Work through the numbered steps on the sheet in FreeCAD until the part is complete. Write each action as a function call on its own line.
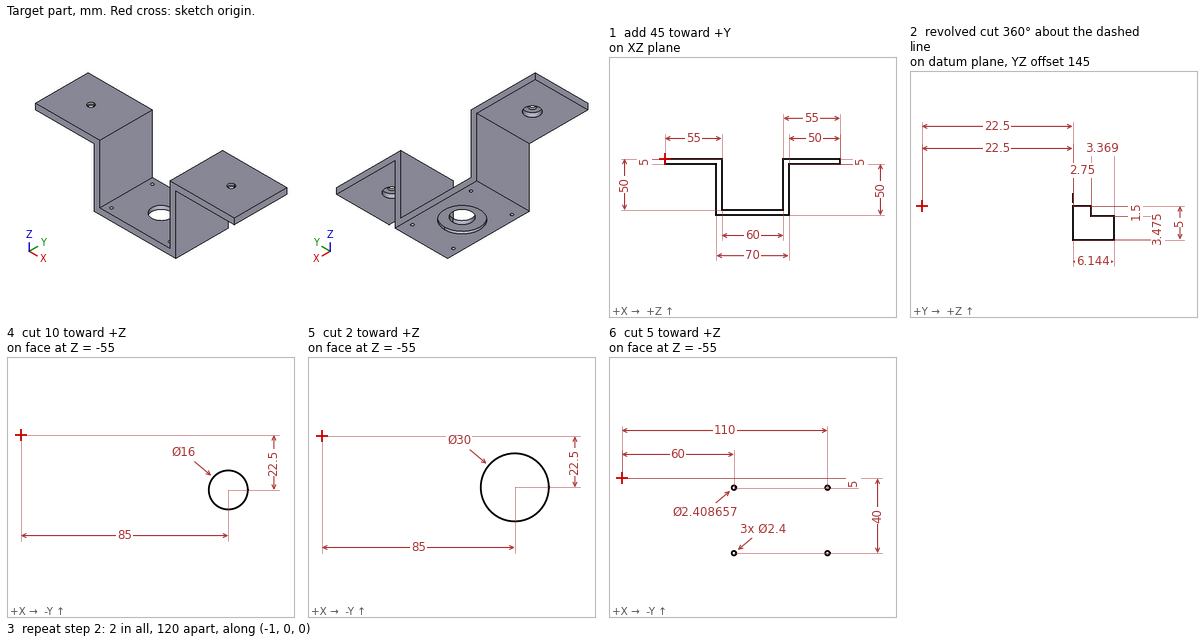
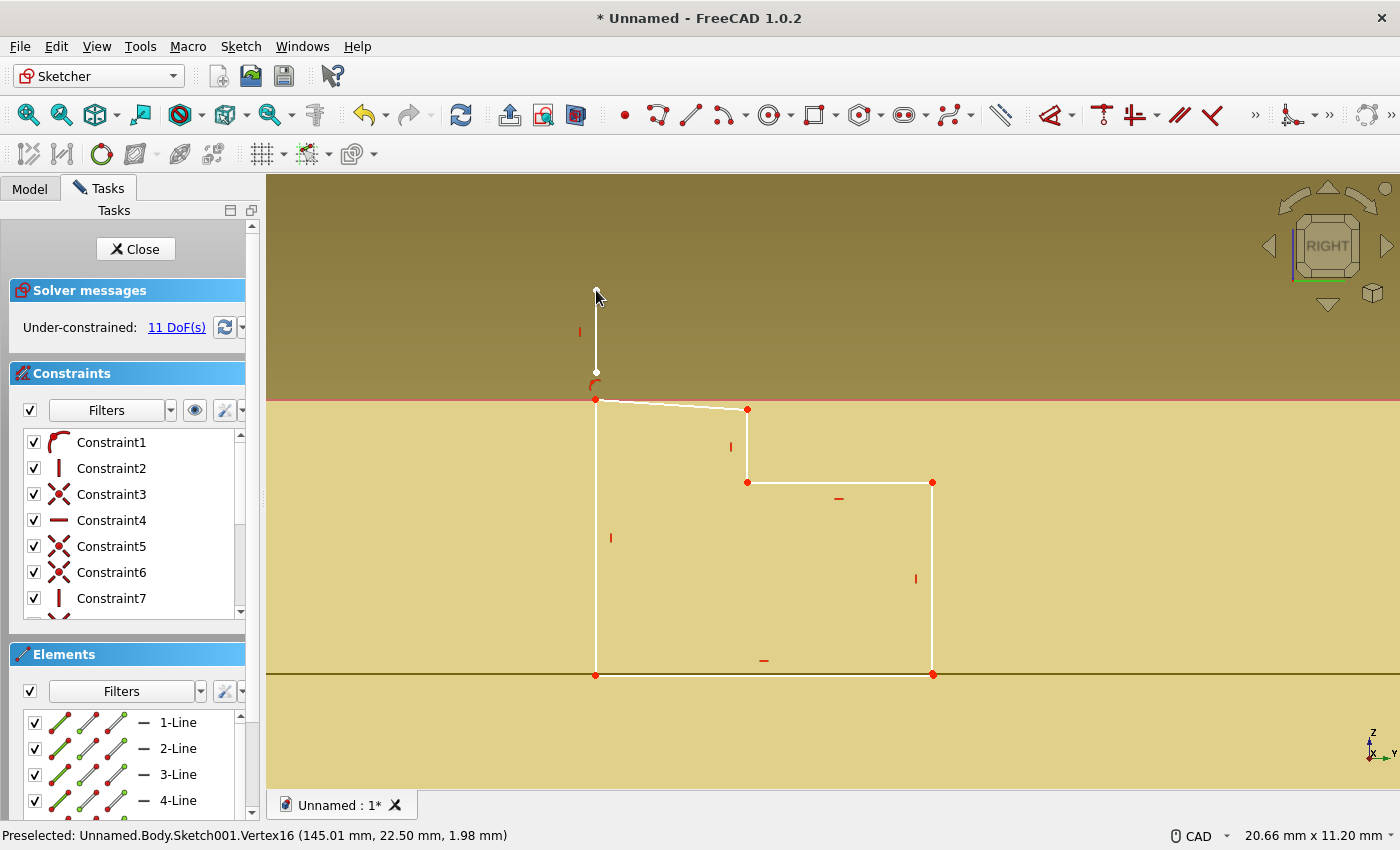
click(596, 348)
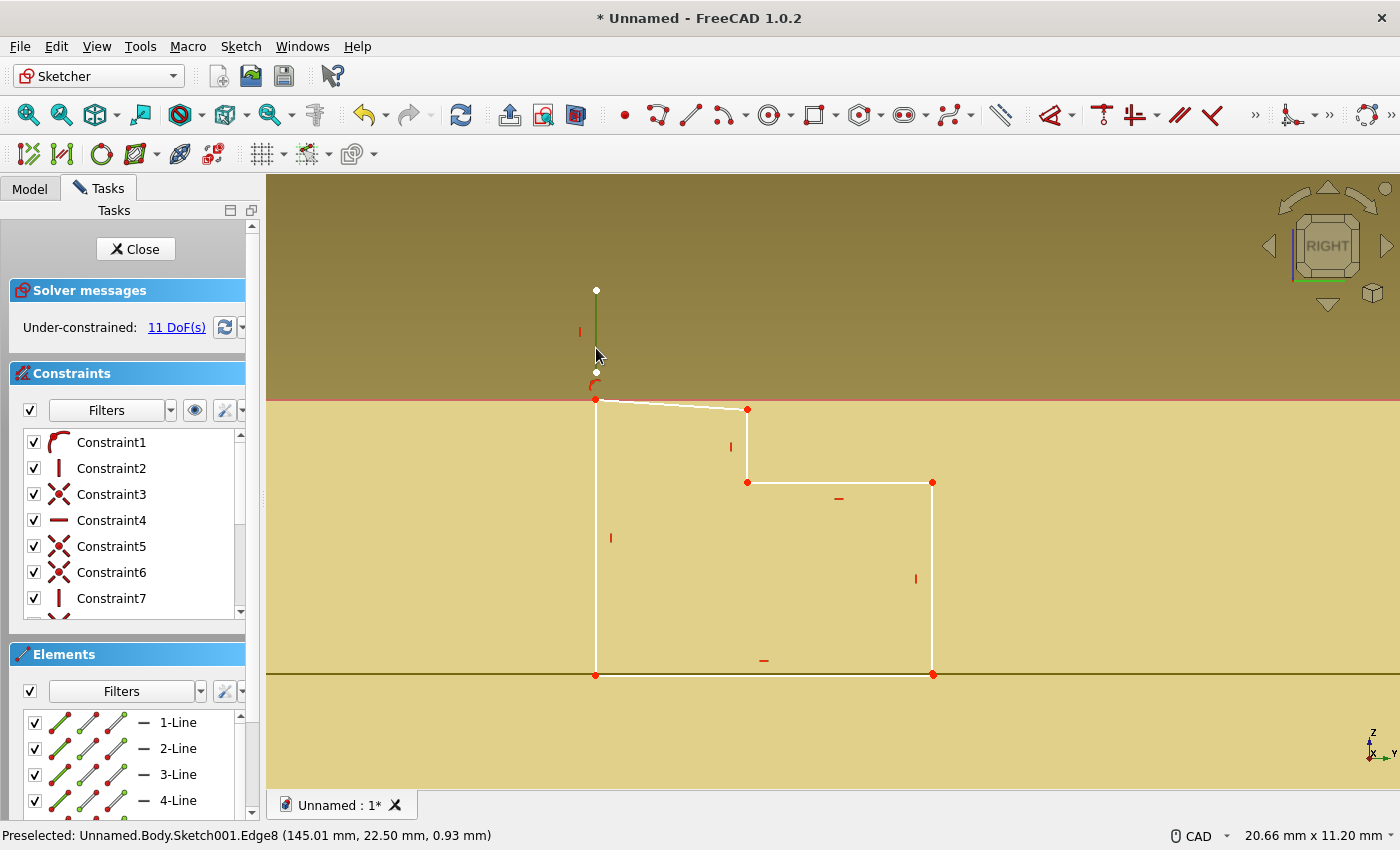
click(1001, 116)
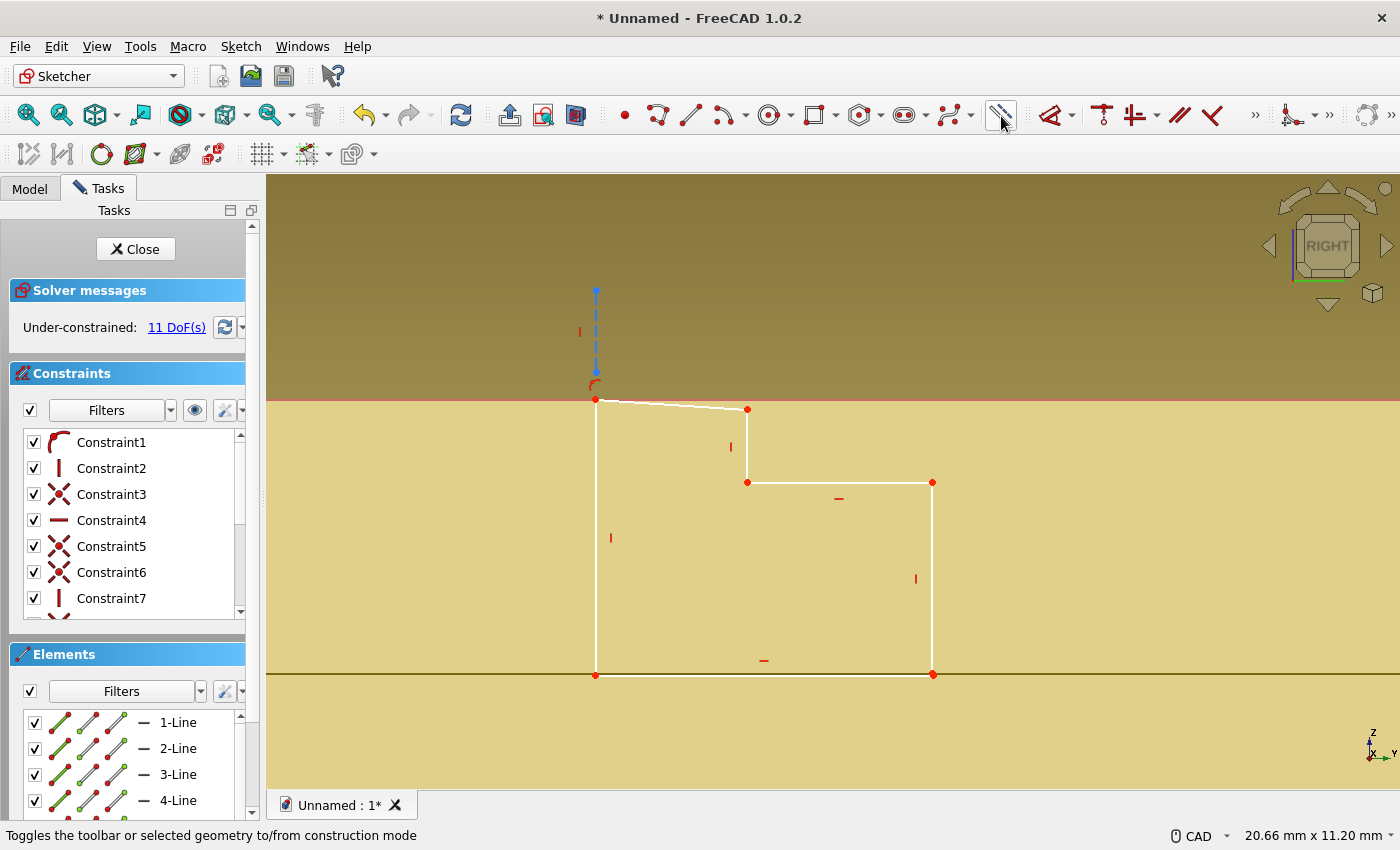
click(641, 403)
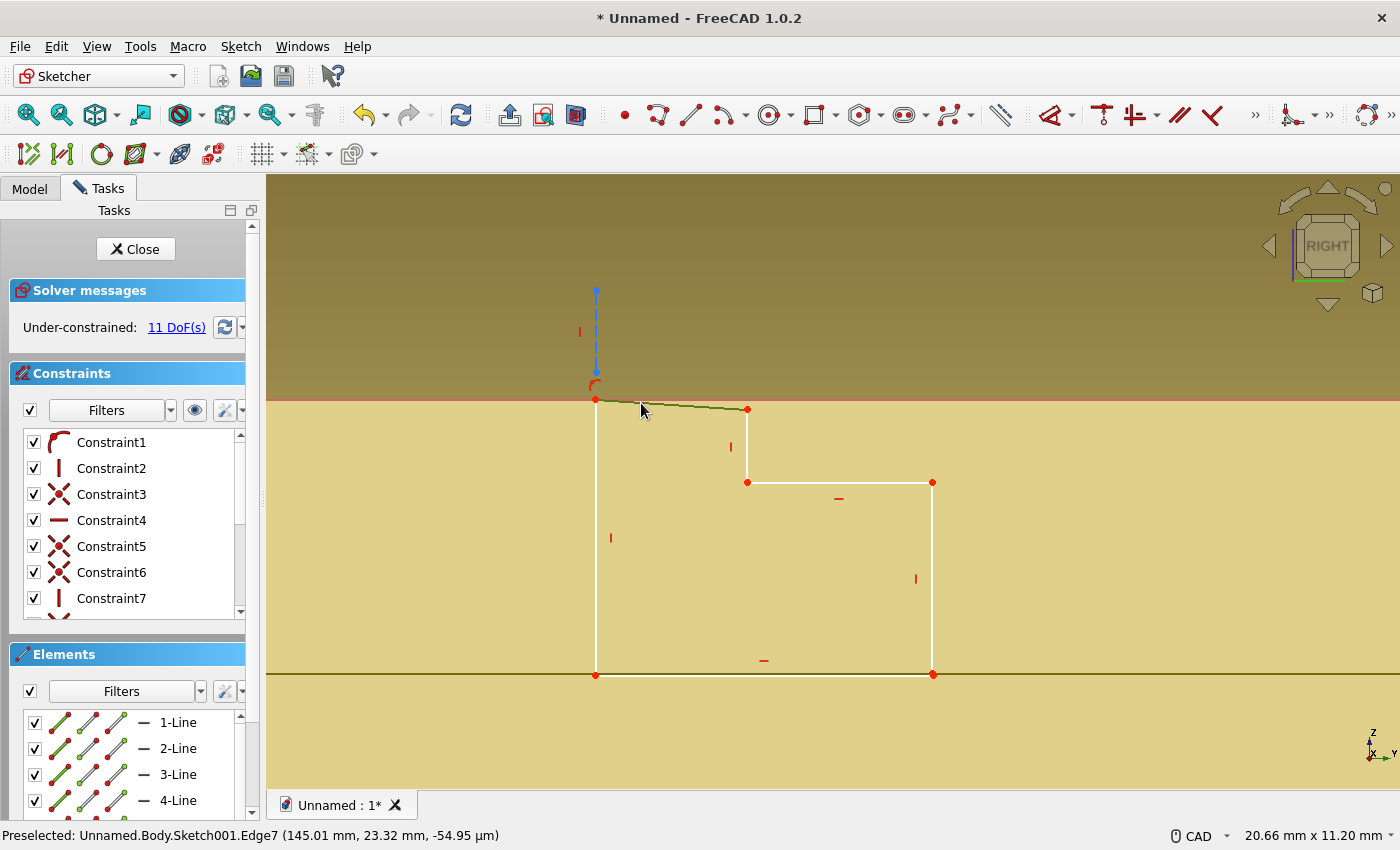
click(1156, 116)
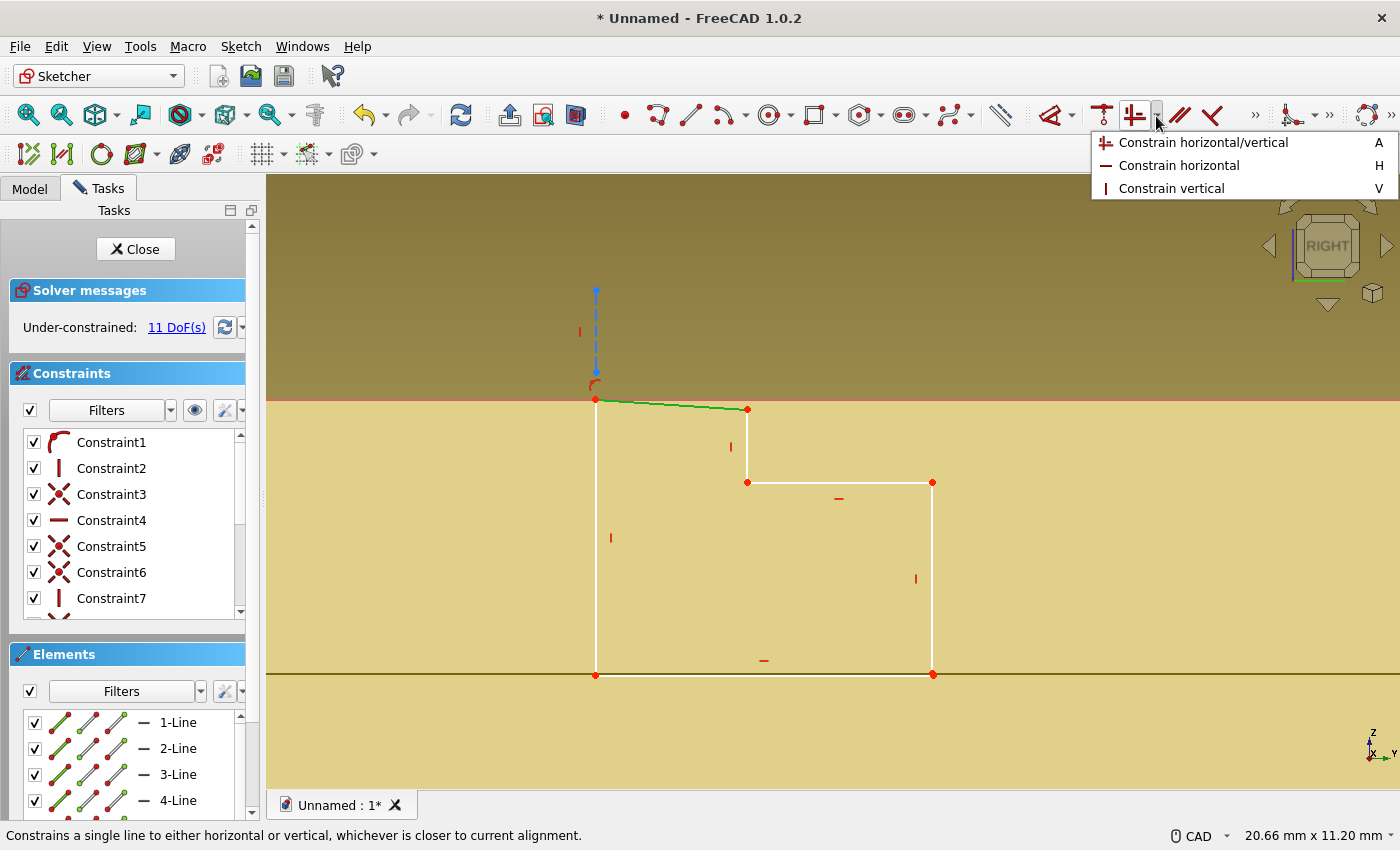
click(1245, 166)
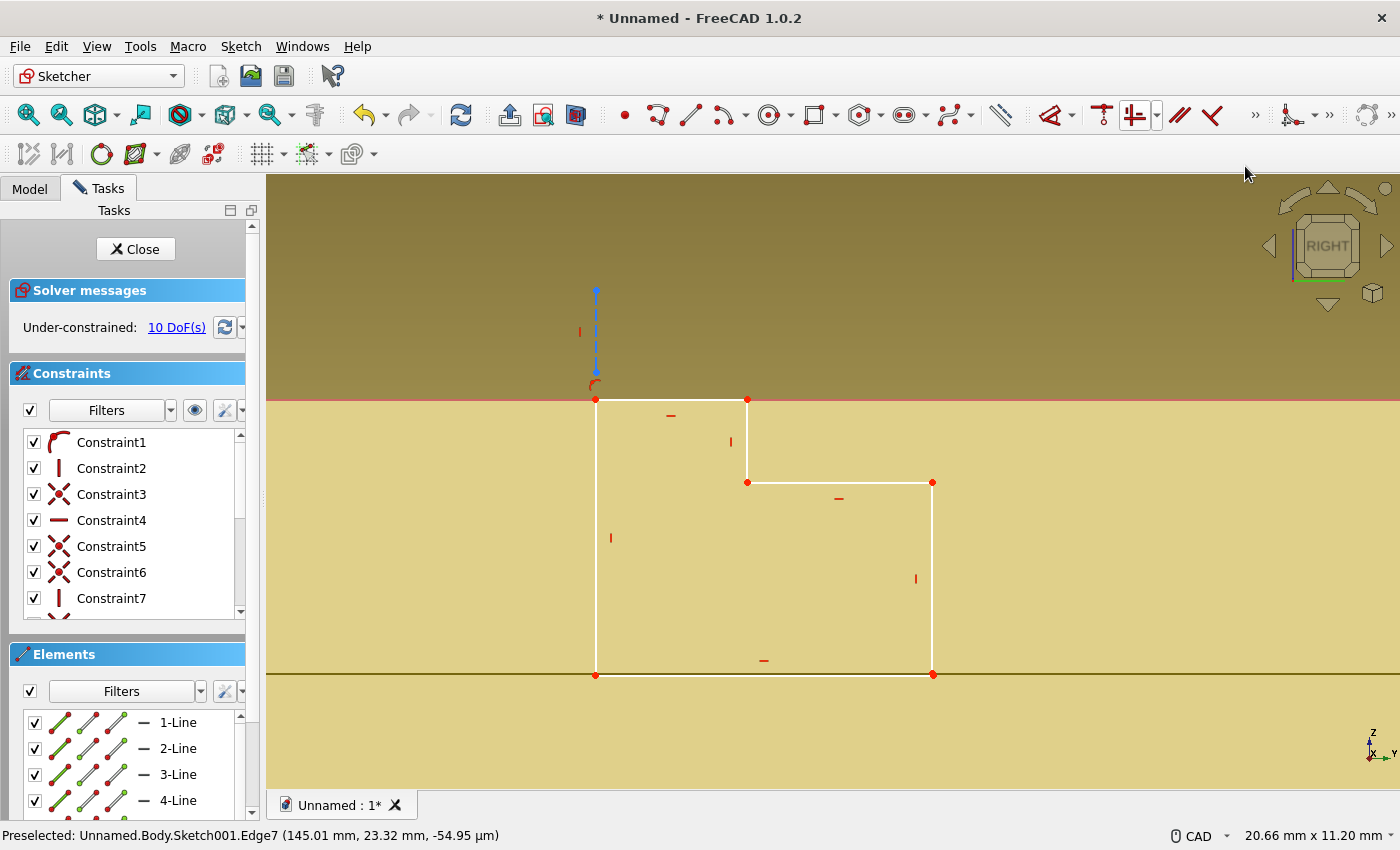
click(1050, 116)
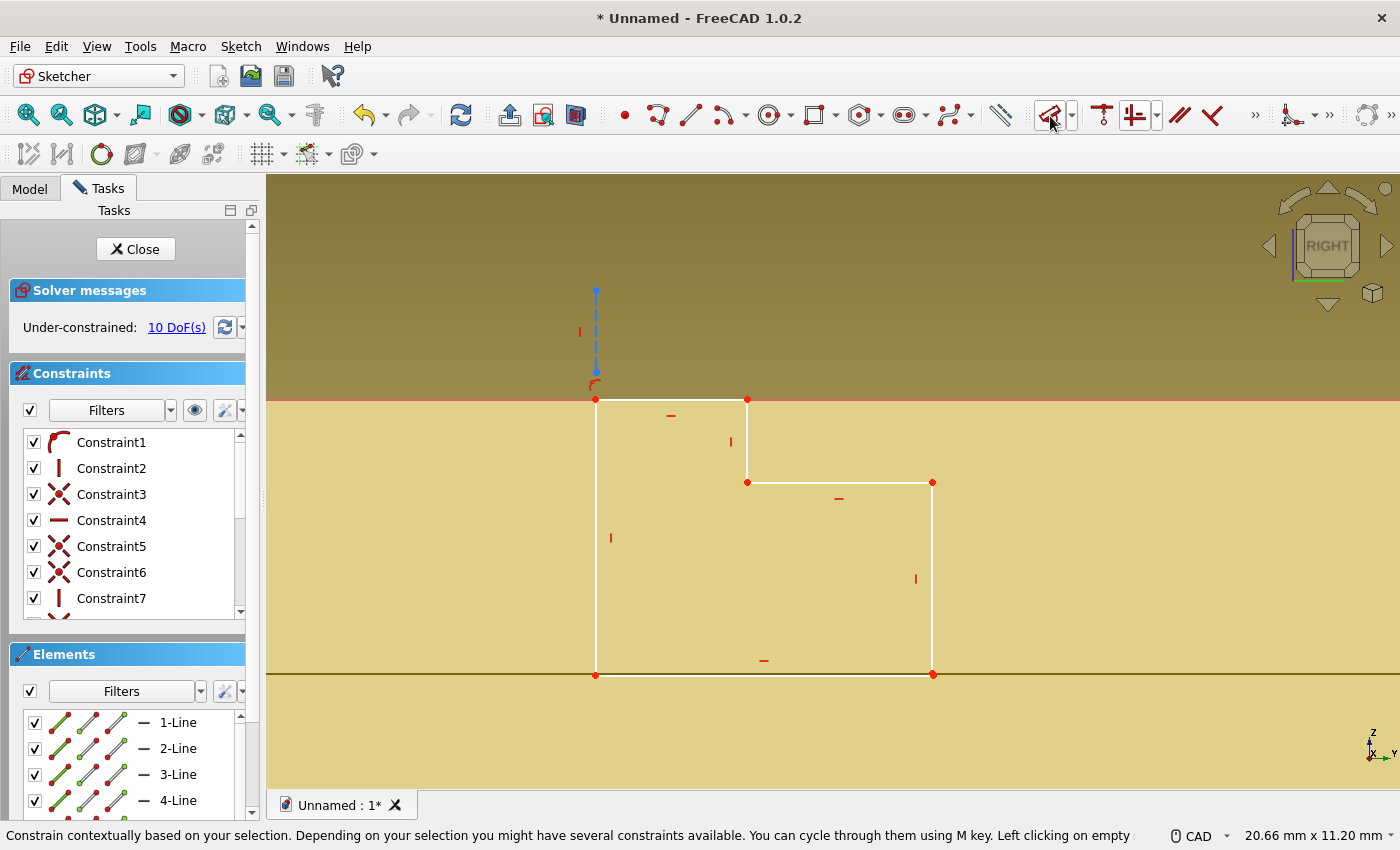
click(596, 483)
click(562, 538)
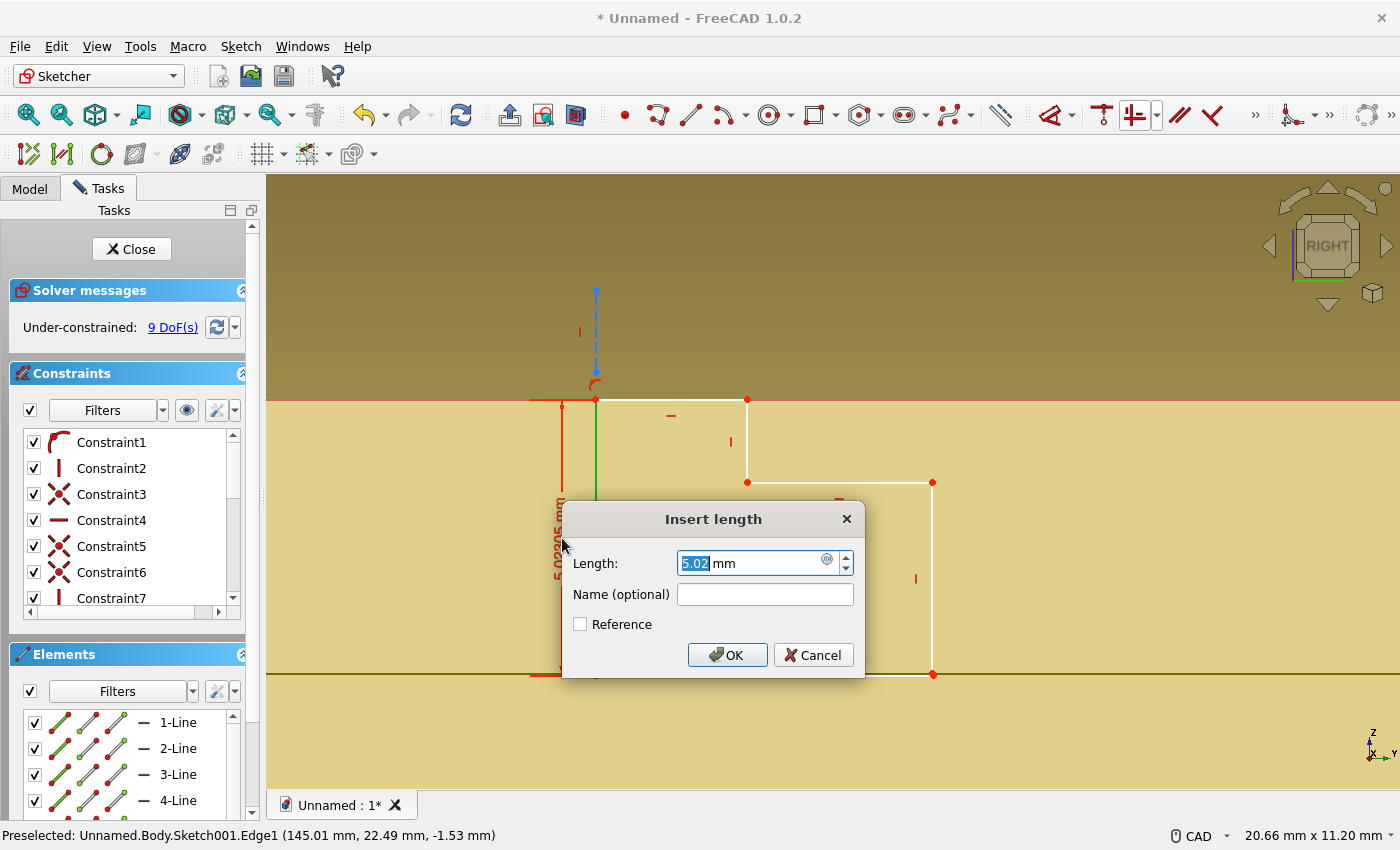
text(5)
key(Return)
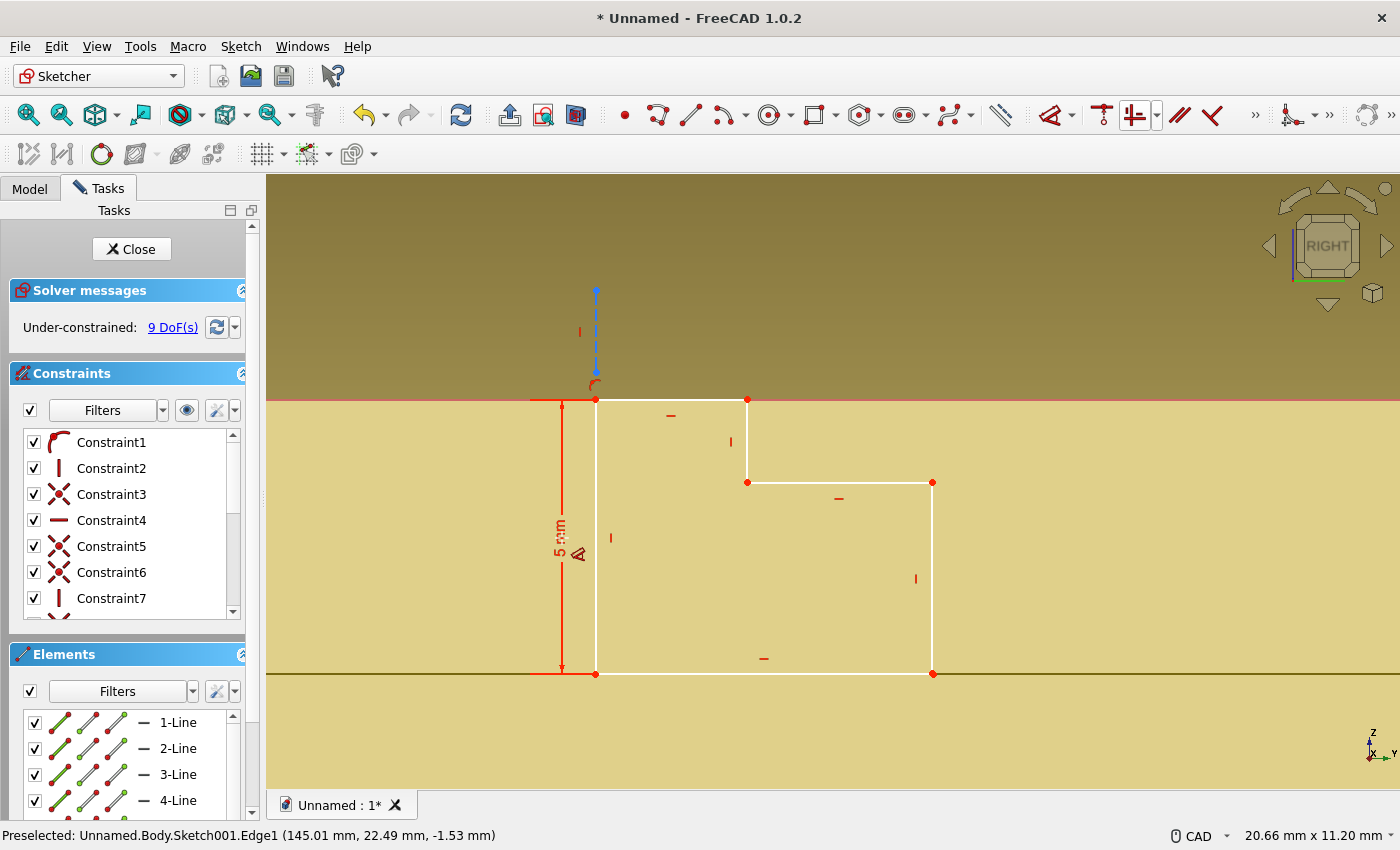
click(747, 458)
click(713, 441)